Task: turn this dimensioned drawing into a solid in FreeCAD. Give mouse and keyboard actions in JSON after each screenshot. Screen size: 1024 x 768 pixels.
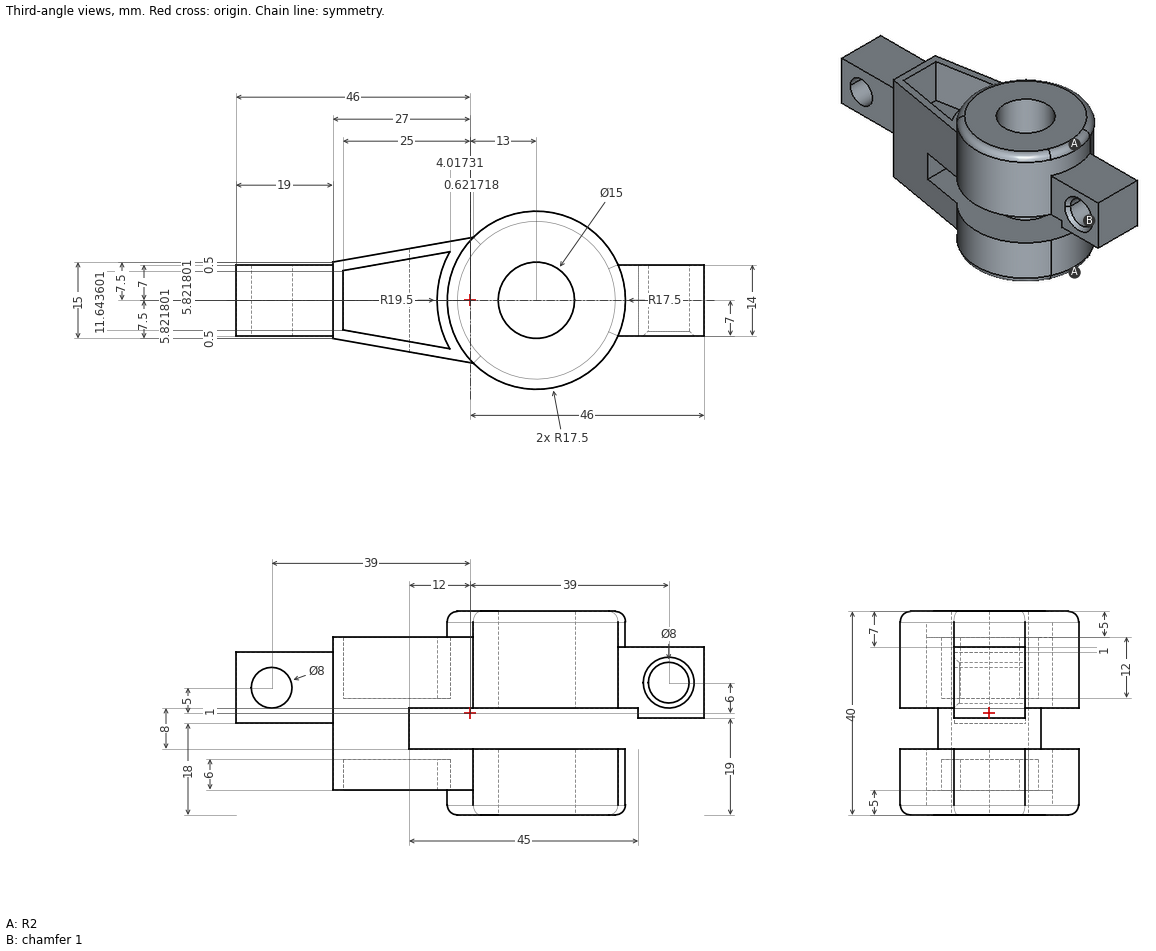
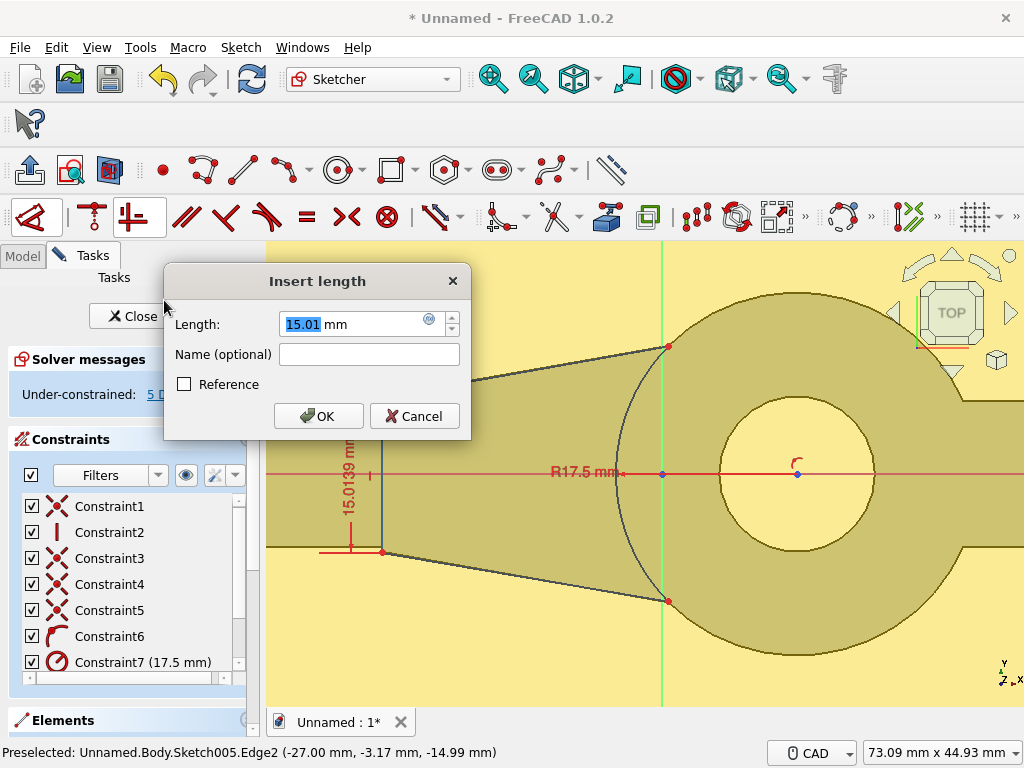
{"action": "type", "text": "15"}
{"action": "key", "text": "Return"}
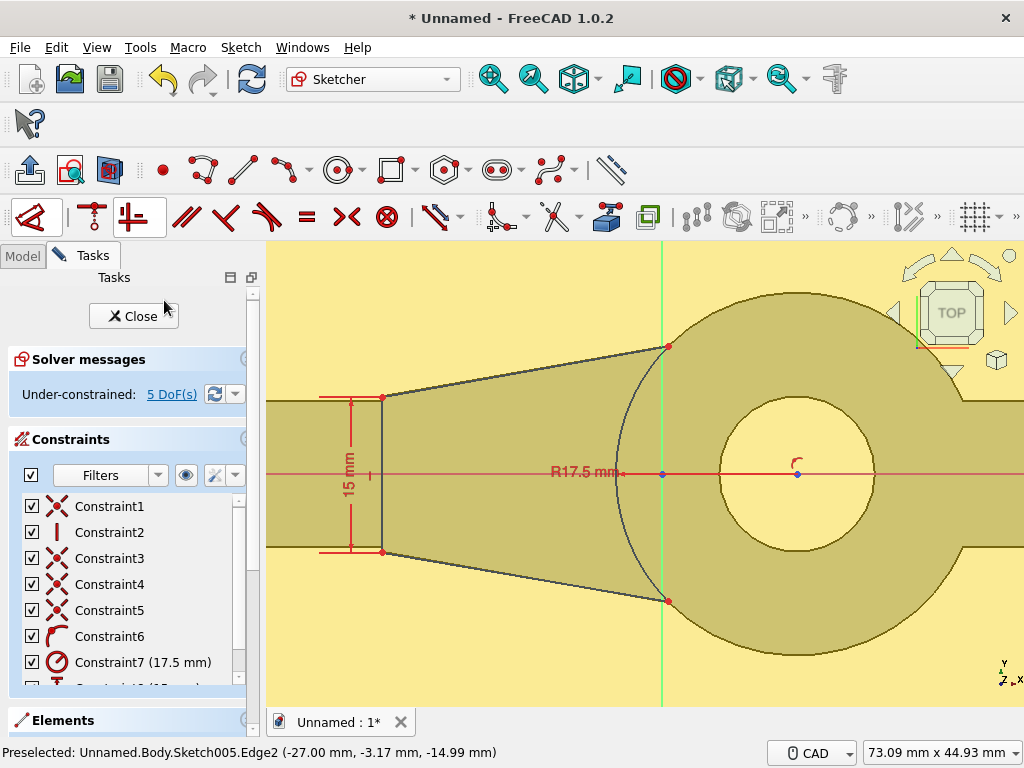
{"action": "left_click", "coordinate": [382, 553]}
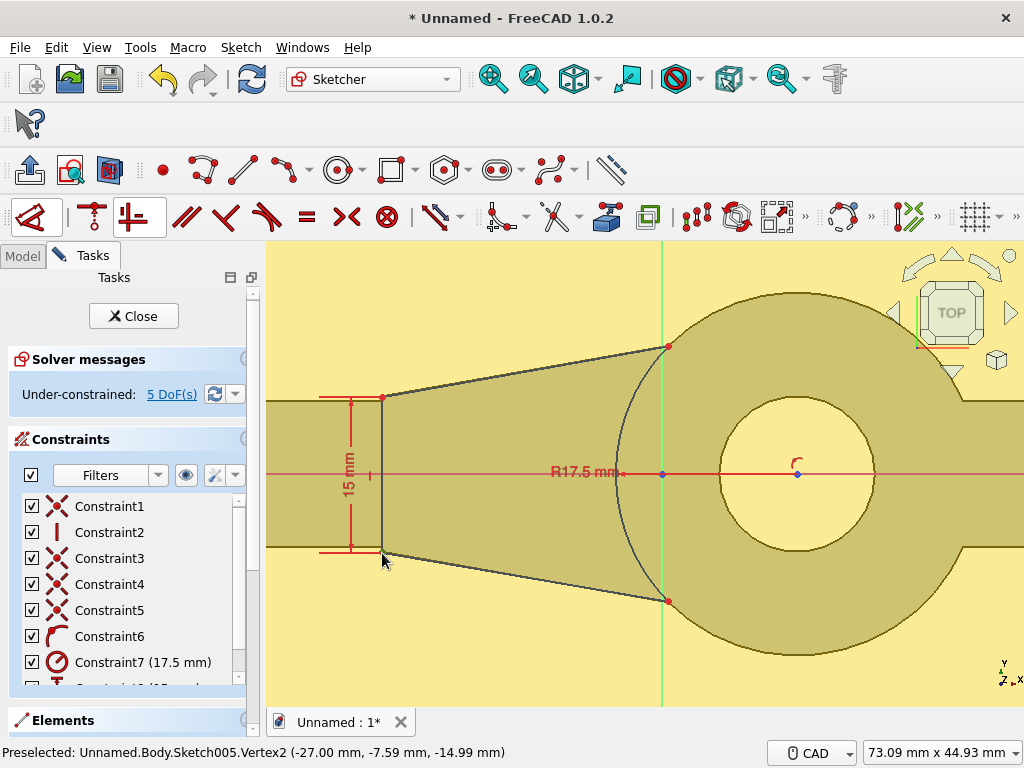
{"action": "left_click", "coordinate": [56, 218]}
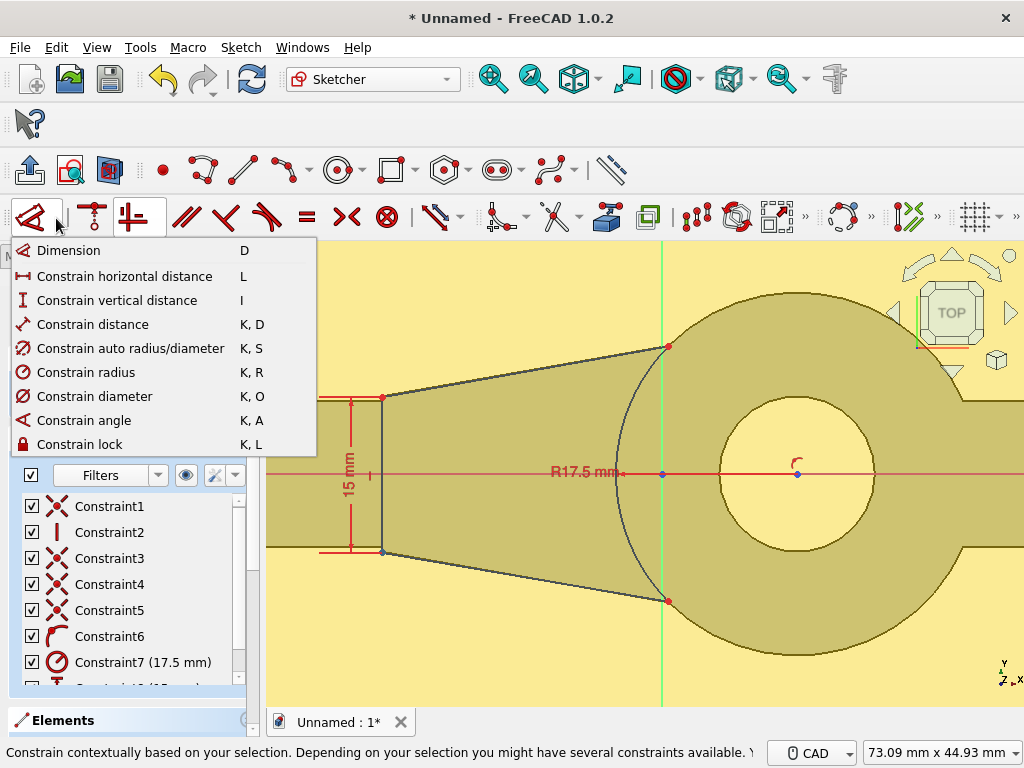
{"action": "left_click", "coordinate": [164, 276]}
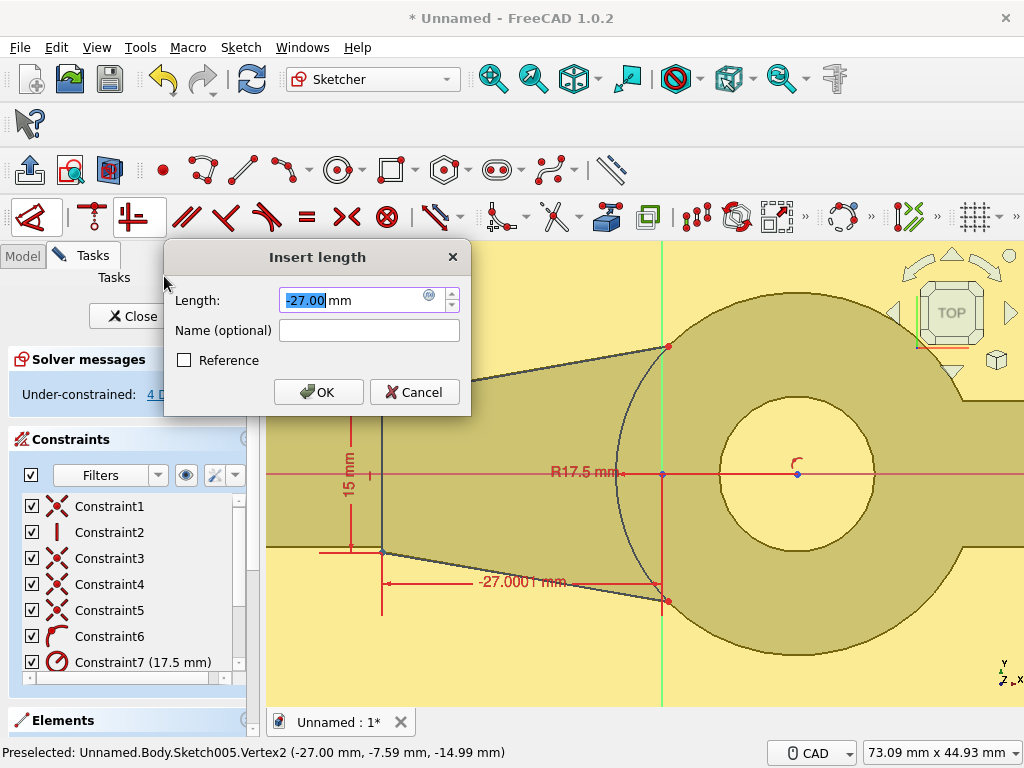
{"action": "type", "text": "-27"}
{"action": "key", "text": "Return"}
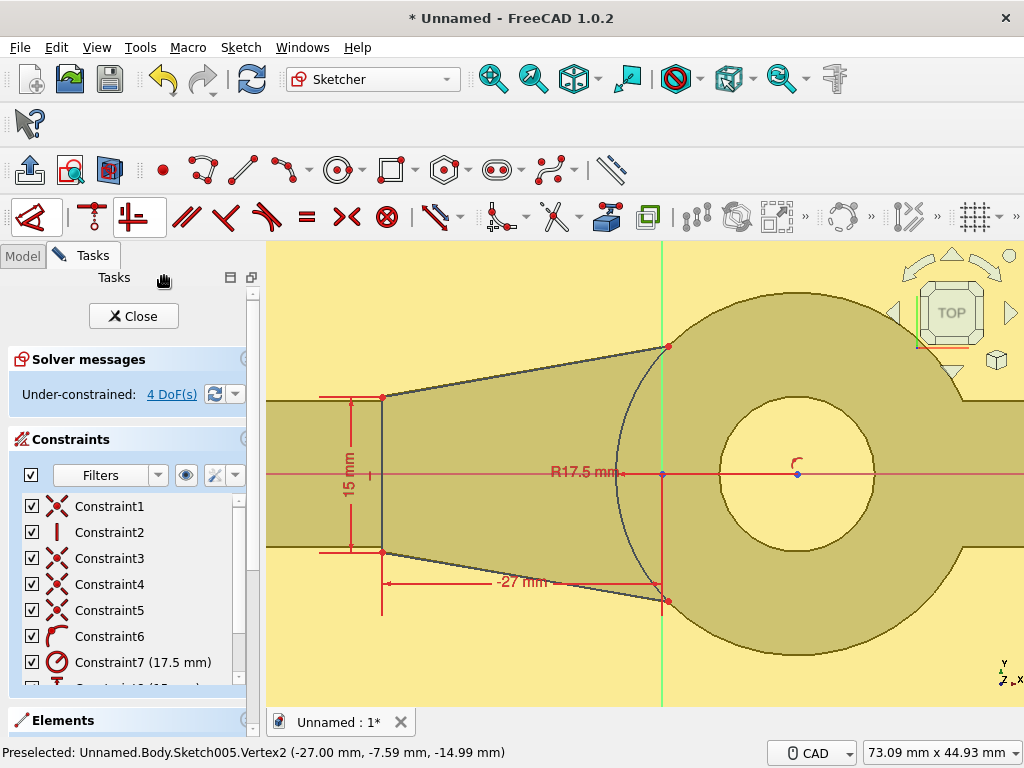
{"action": "left_click", "coordinate": [798, 474]}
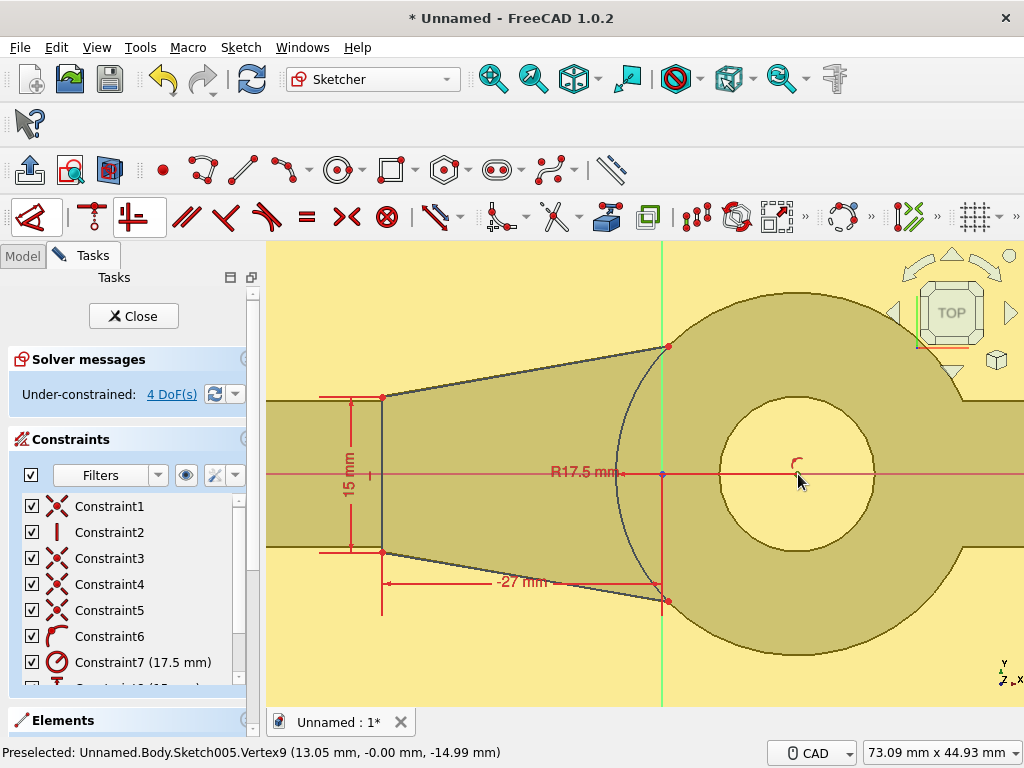
{"action": "key", "text": "l"}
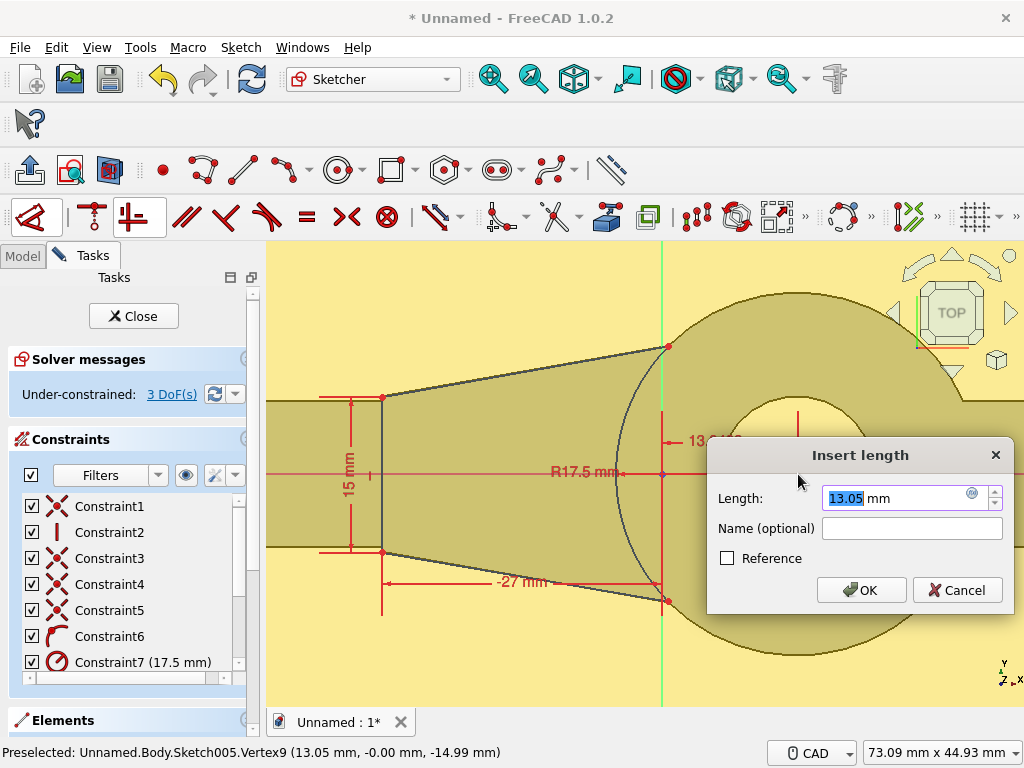
{"action": "type", "text": "13"}
{"action": "key", "text": "Return"}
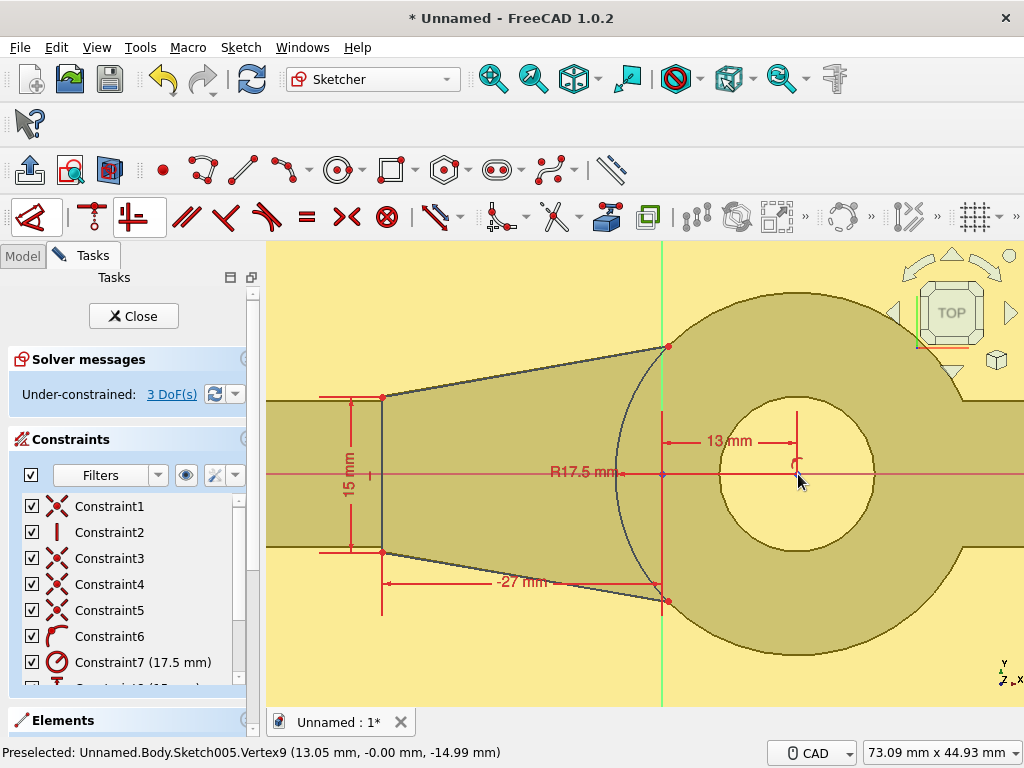
{"action": "left_click", "coordinate": [382, 553]}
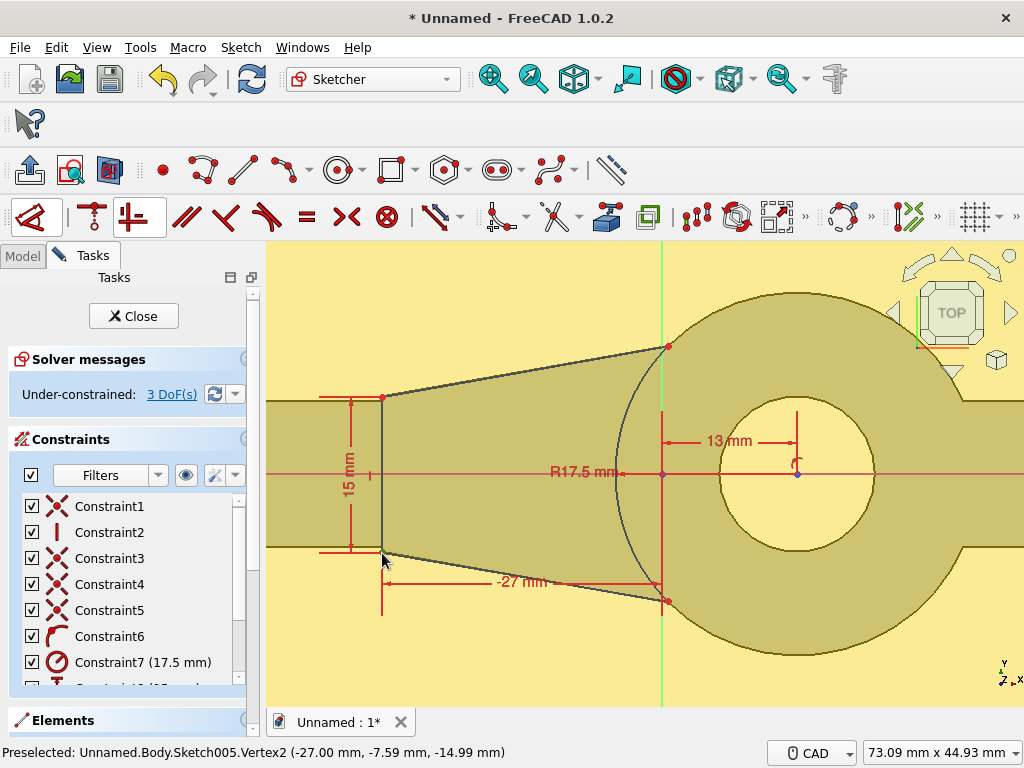
{"action": "left_click", "coordinate": [56, 218]}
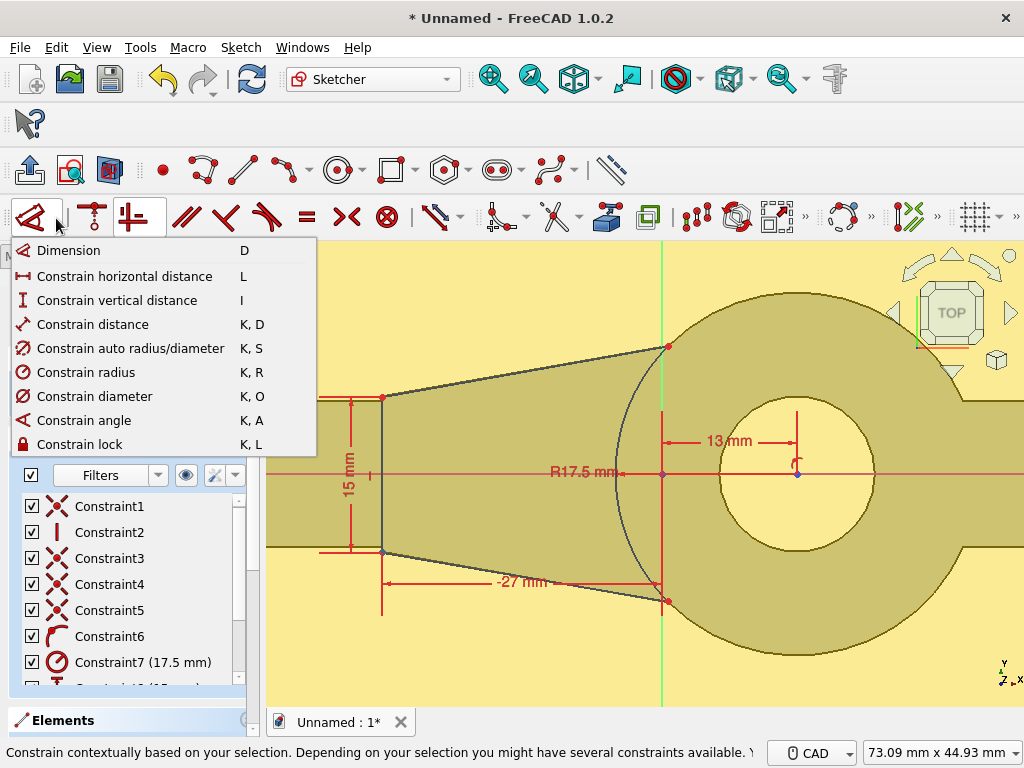
{"action": "left_click", "coordinate": [164, 300]}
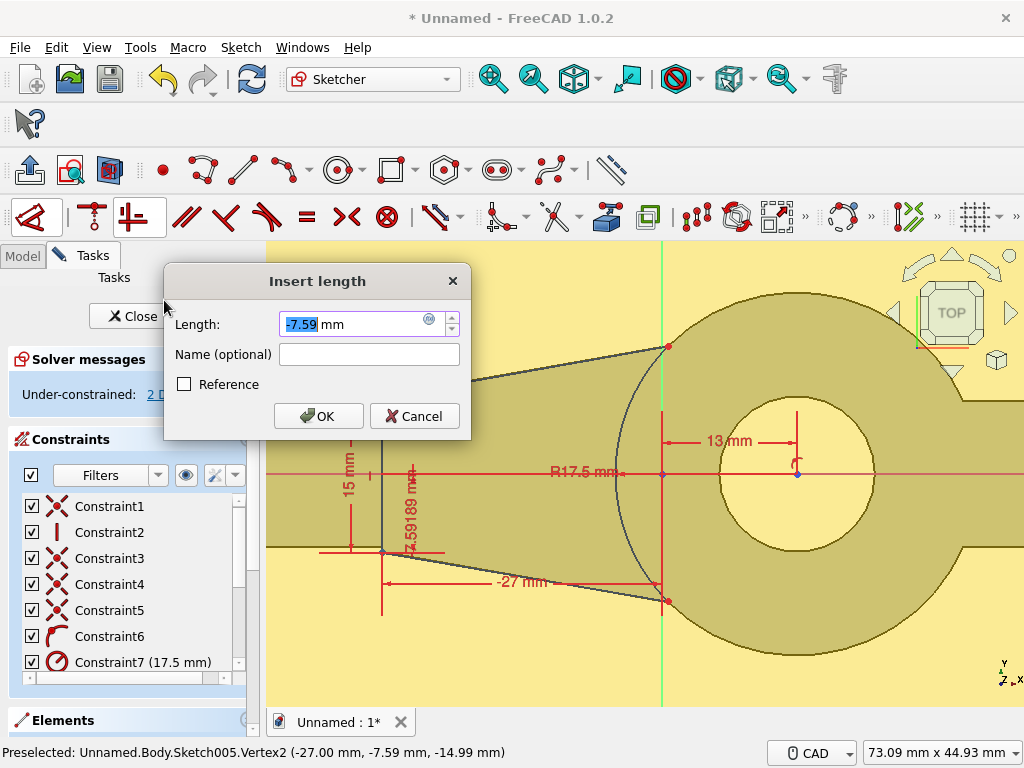
{"action": "type", "text": "-7.5"}
{"action": "key", "text": "Return"}